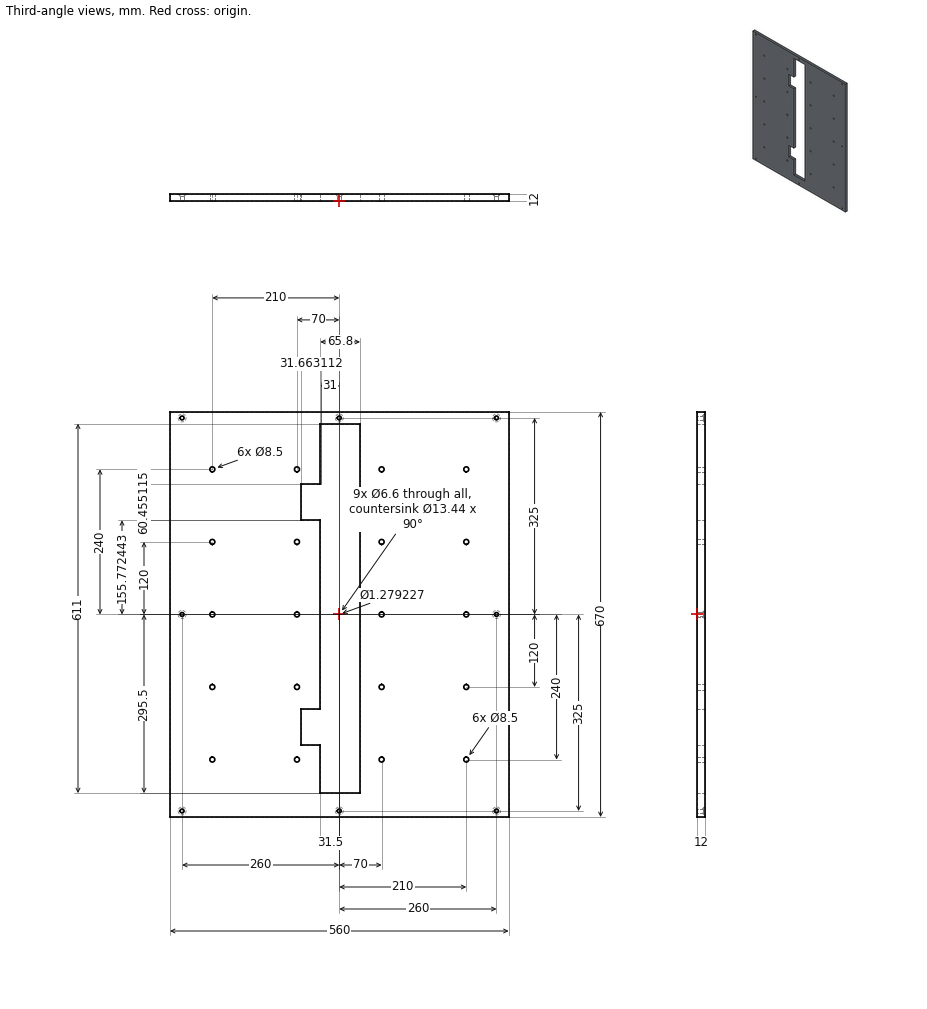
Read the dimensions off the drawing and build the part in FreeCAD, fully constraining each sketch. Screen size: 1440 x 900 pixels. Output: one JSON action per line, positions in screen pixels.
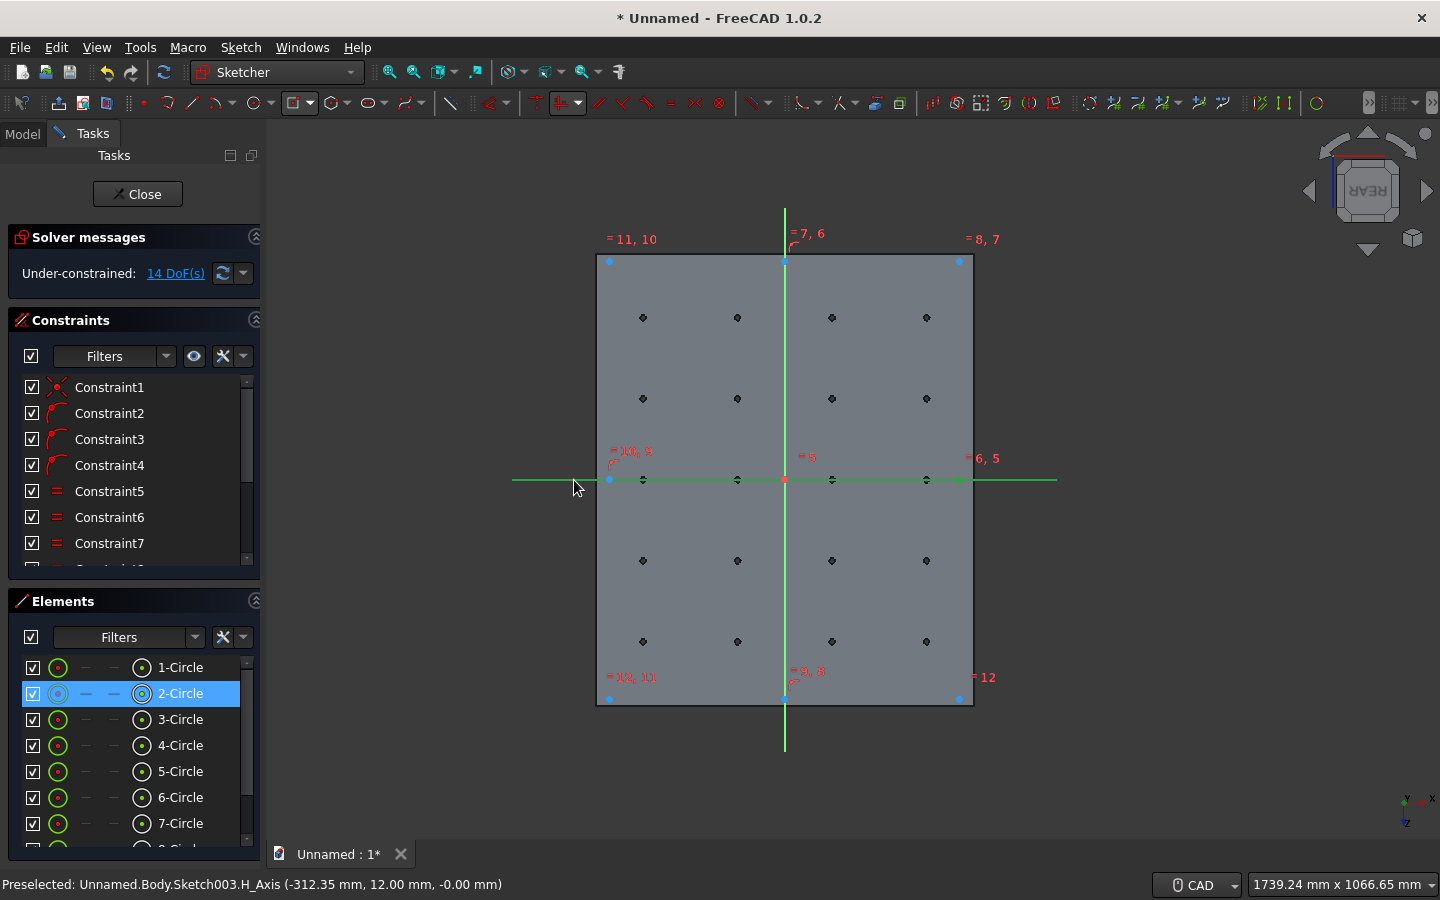
{"action": "left_click", "coordinate": [536, 104]}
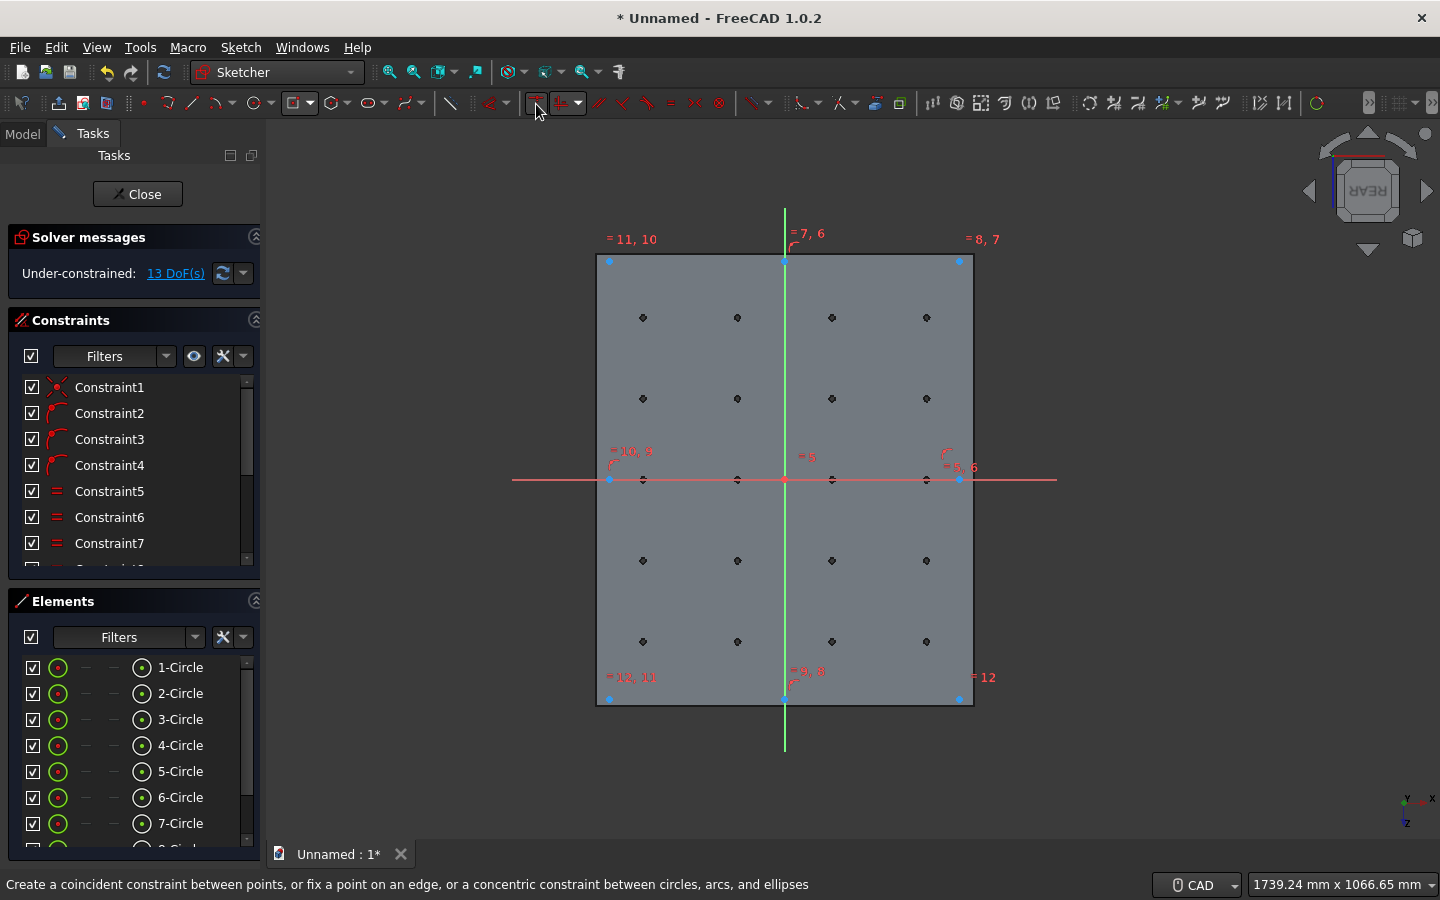
{"action": "left_click", "coordinate": [960, 480]}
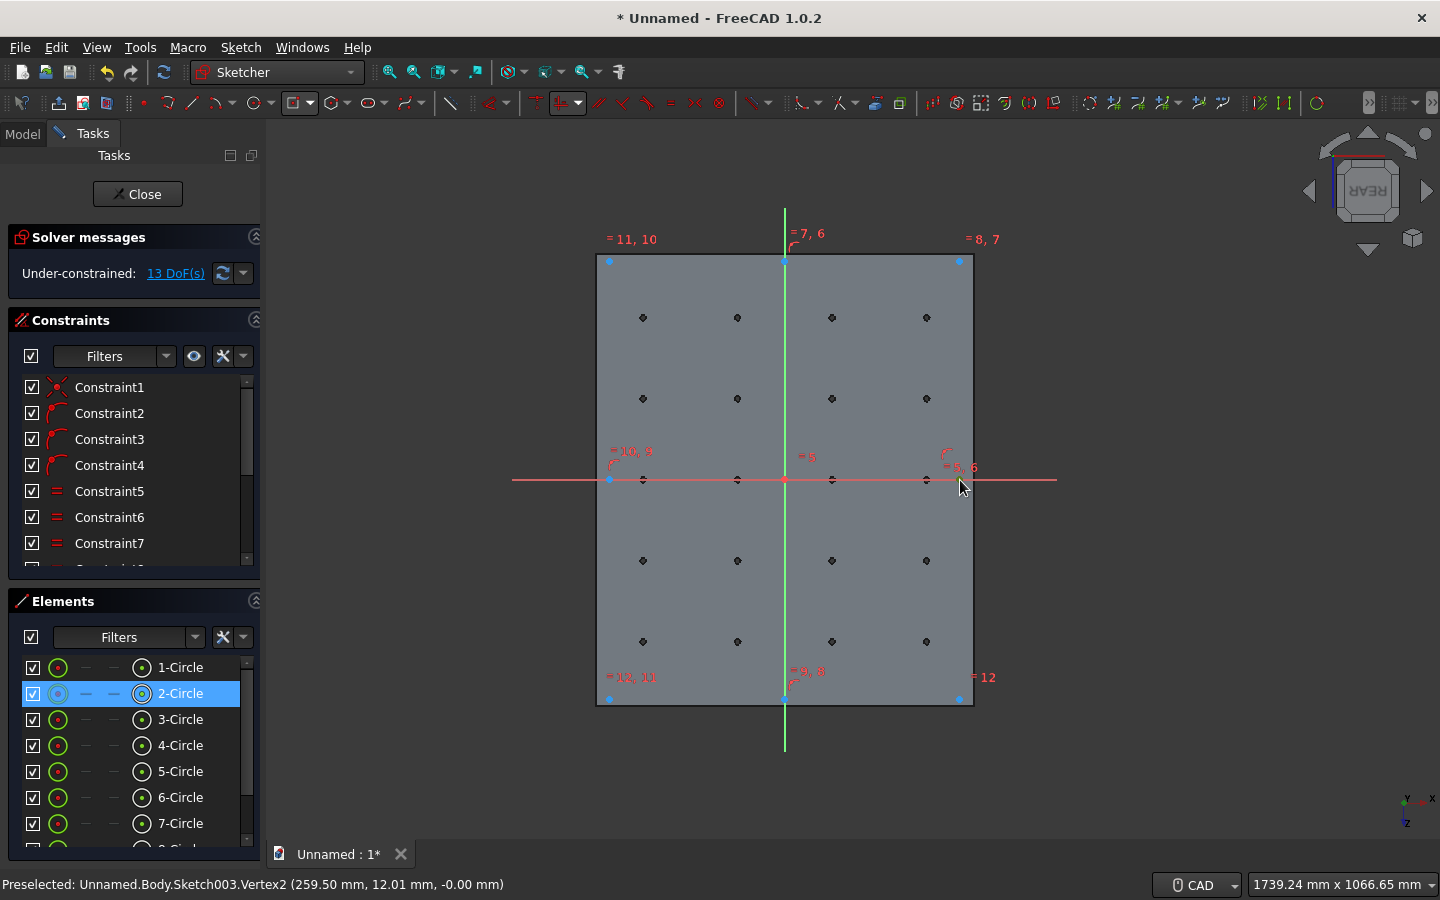
{"action": "left_click", "coordinate": [960, 262]}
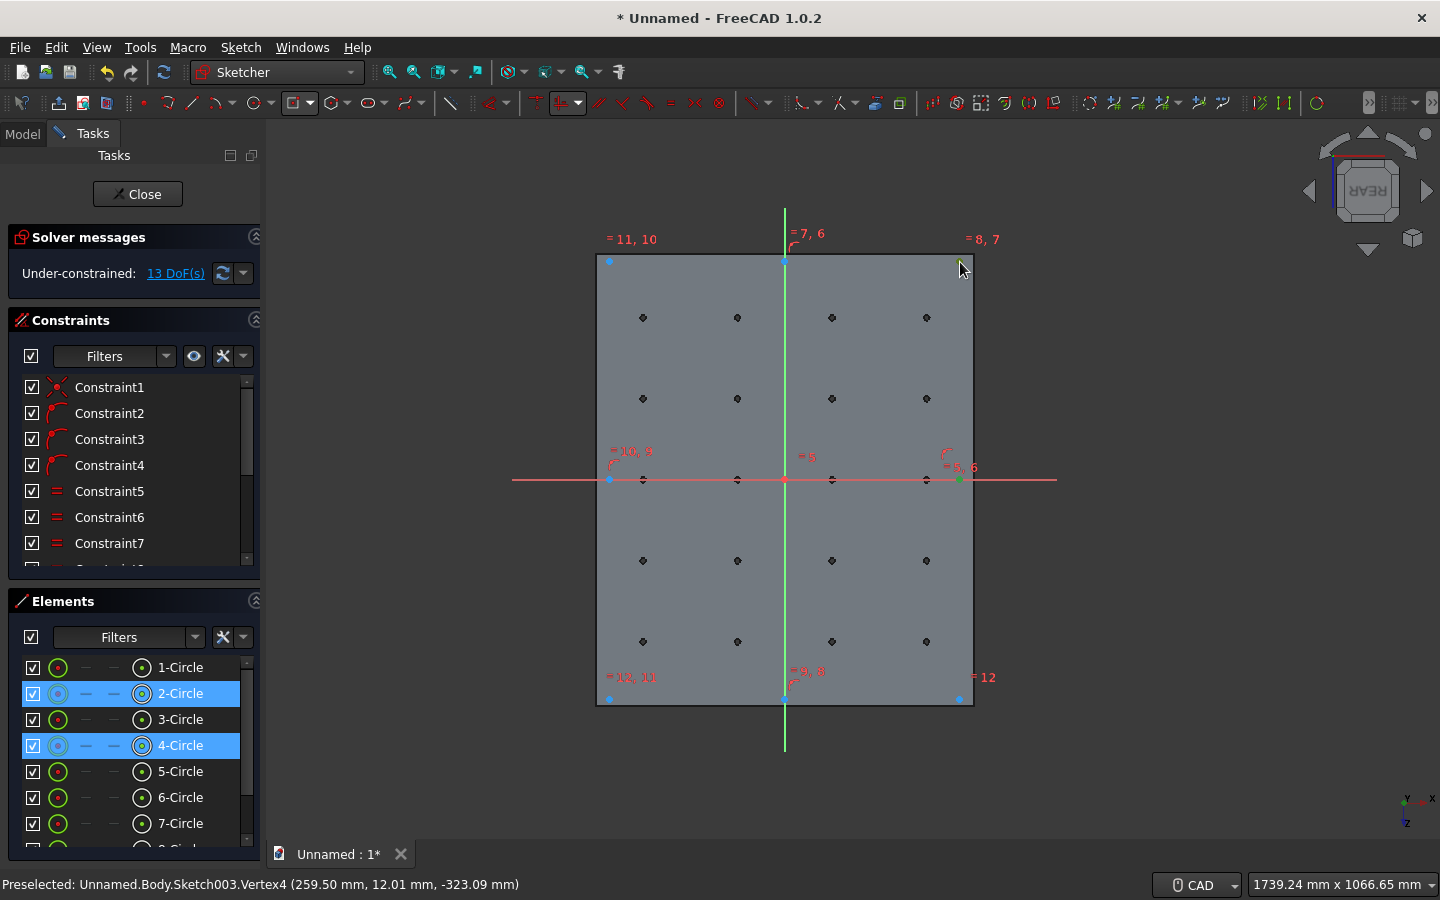
{"action": "left_click", "coordinate": [580, 104]}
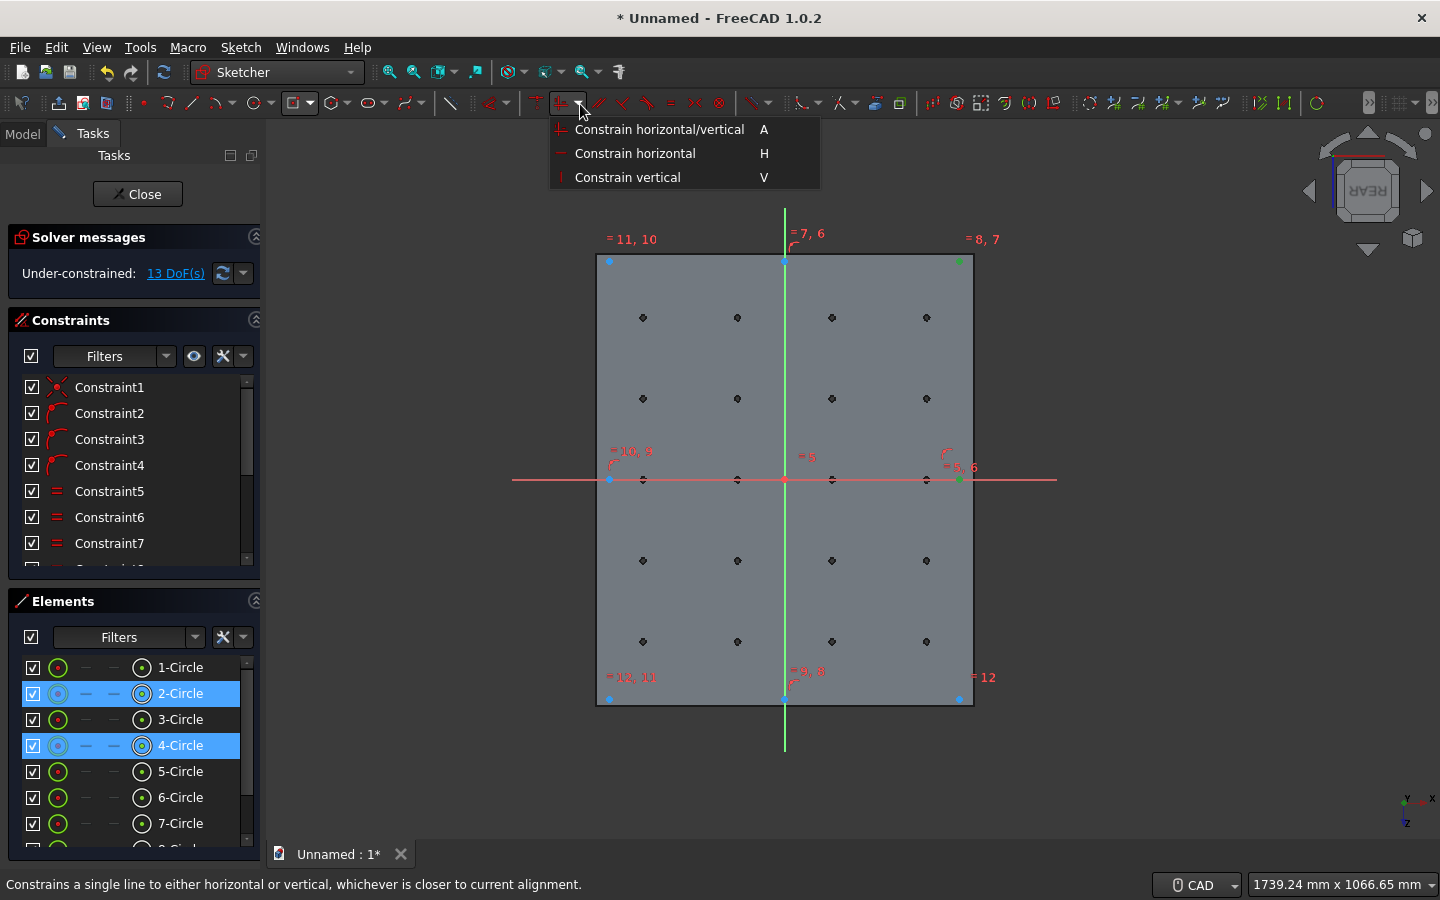
{"action": "left_click", "coordinate": [685, 177]}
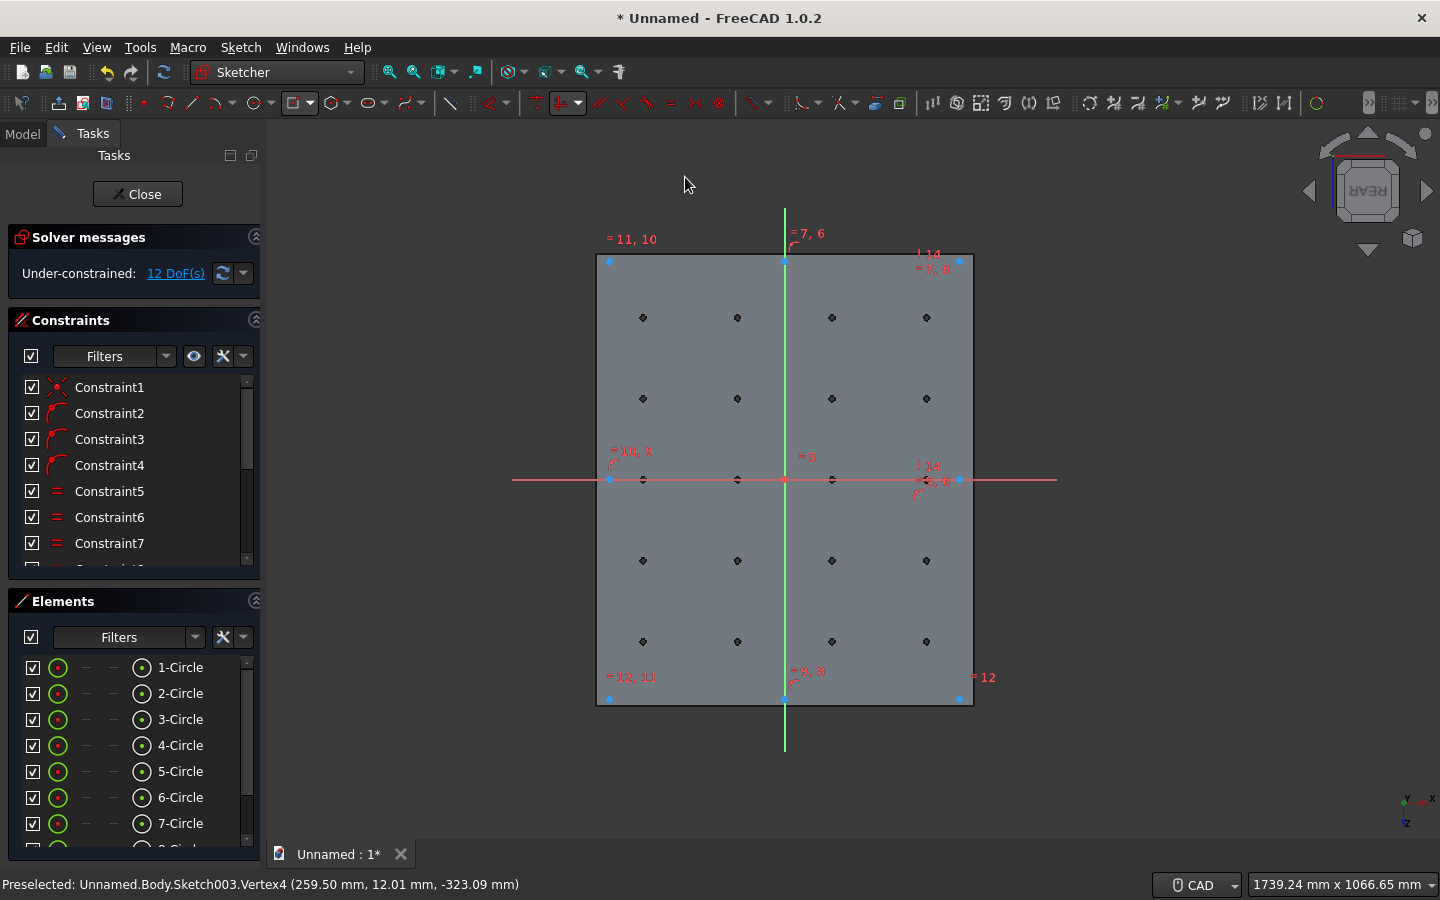
{"action": "left_click", "coordinate": [785, 262]}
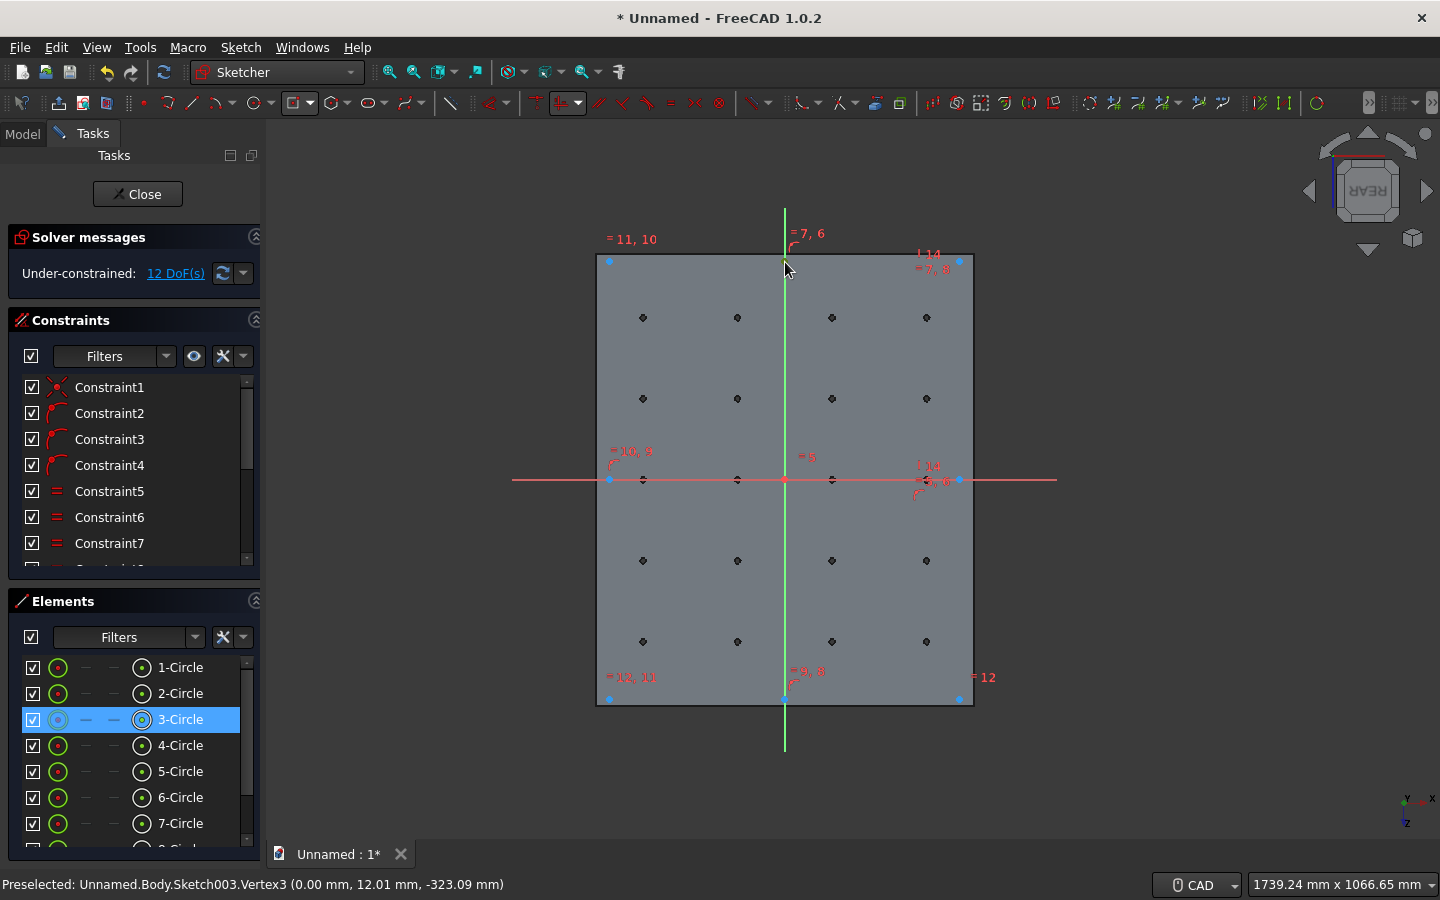
{"action": "left_click", "coordinate": [960, 262]}